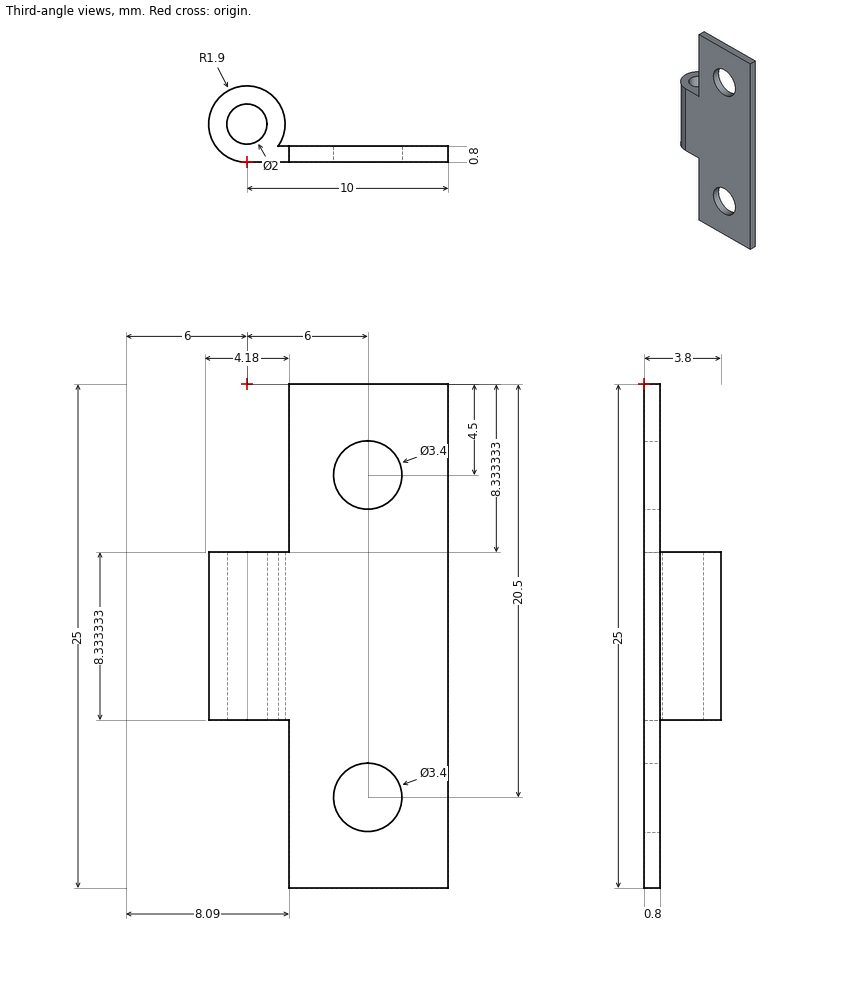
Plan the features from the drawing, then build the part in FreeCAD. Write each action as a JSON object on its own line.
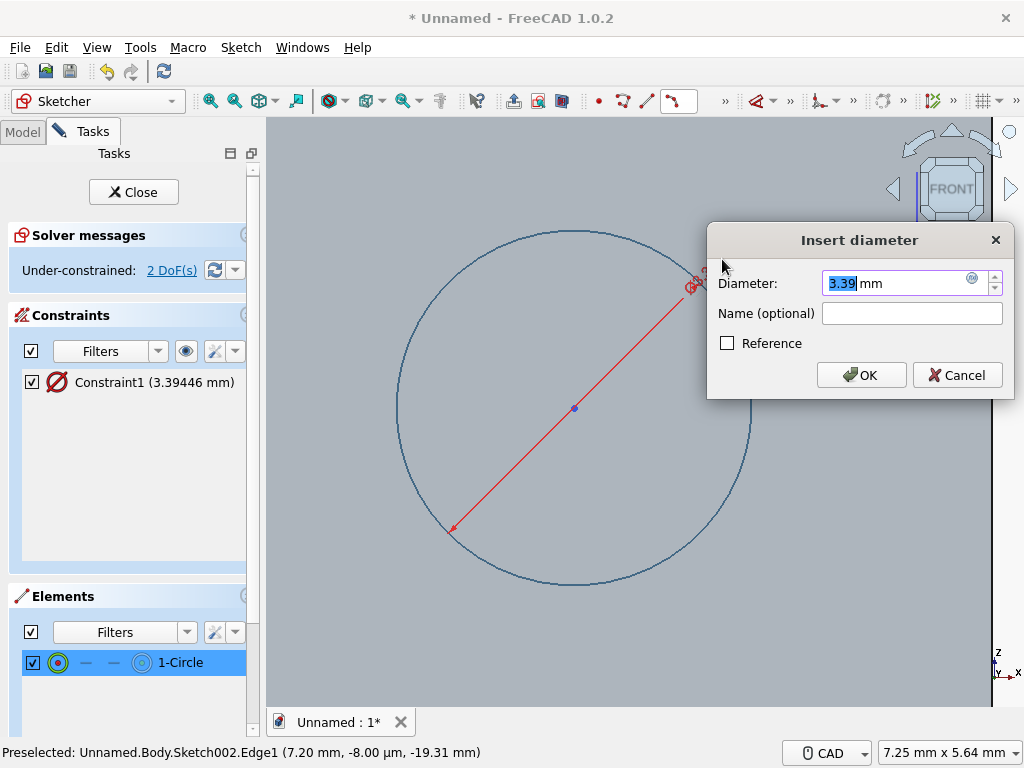
{"action": "type", "text": "3.4"}
{"action": "key", "text": "Return"}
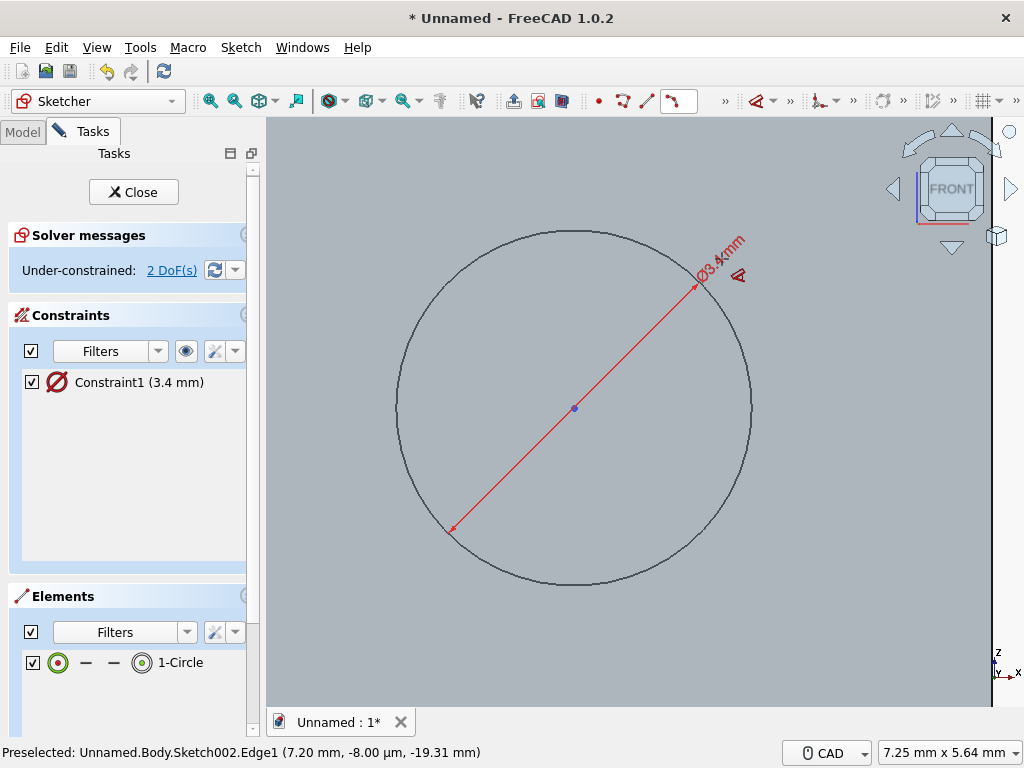
{"action": "left_click", "coordinate": [574, 408]}
{"action": "left_click", "coordinate": [434, 442]}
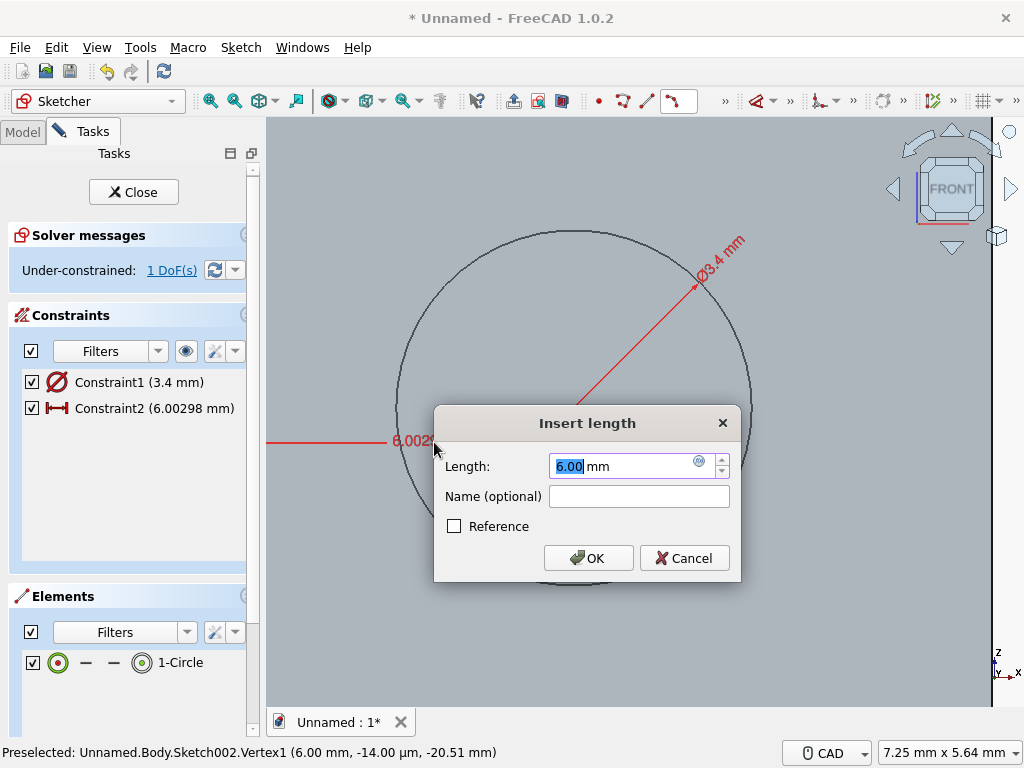
{"action": "type", "text": "6"}
{"action": "key", "text": "Return"}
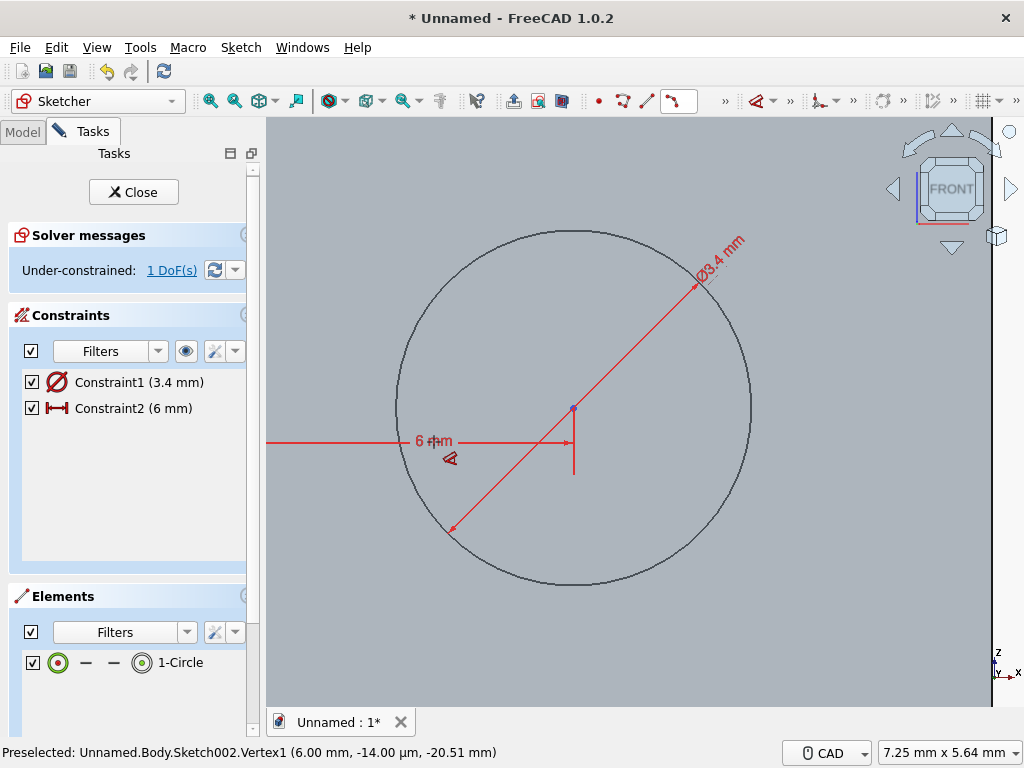
{"action": "left_click", "coordinate": [574, 408]}
{"action": "left_click", "coordinate": [608, 277]}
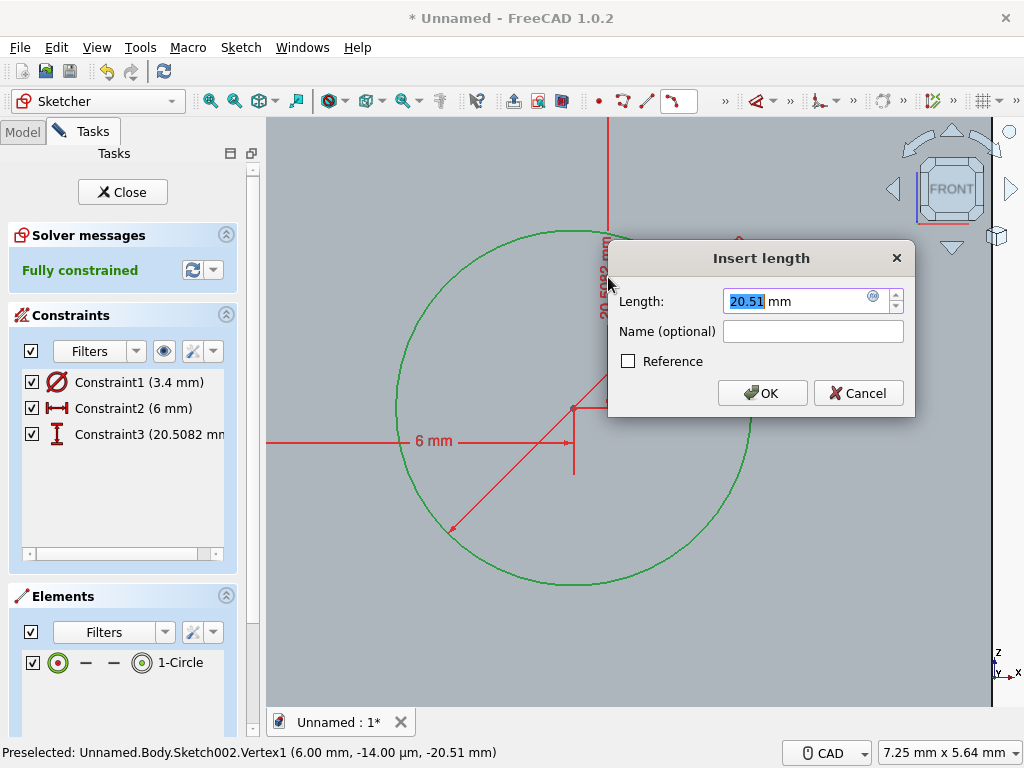
{"action": "type", "text": "20.5"}
{"action": "key", "text": "Return"}
{"action": "key", "text": "Escape"}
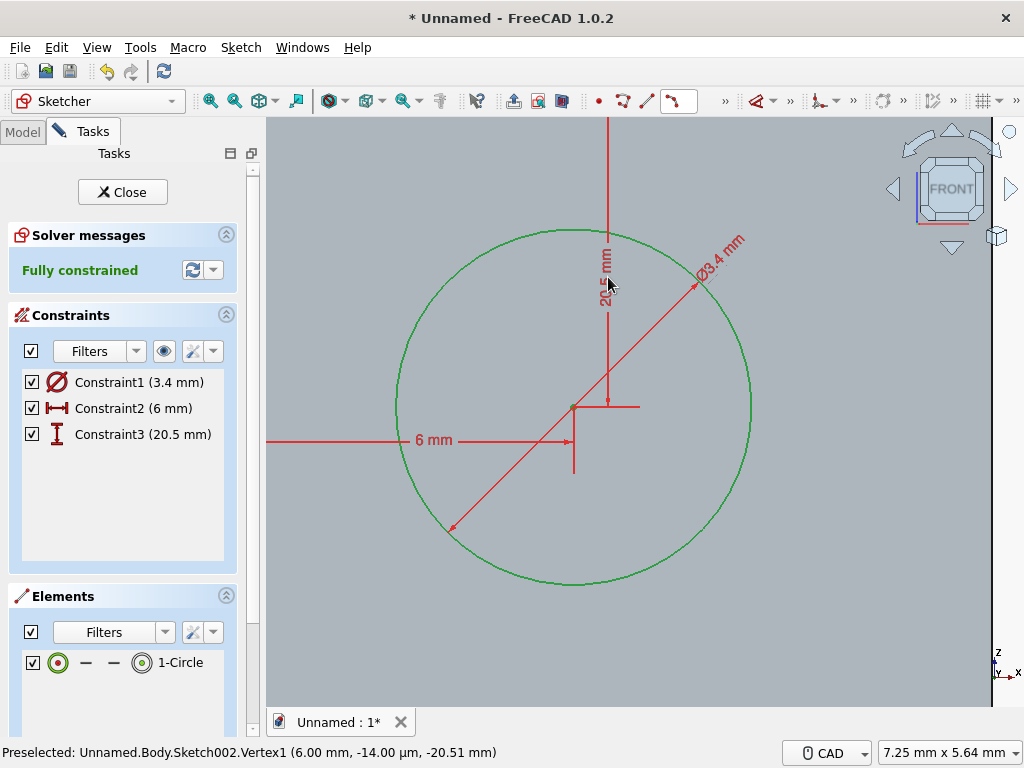
{"action": "left_click", "coordinate": [123, 192]}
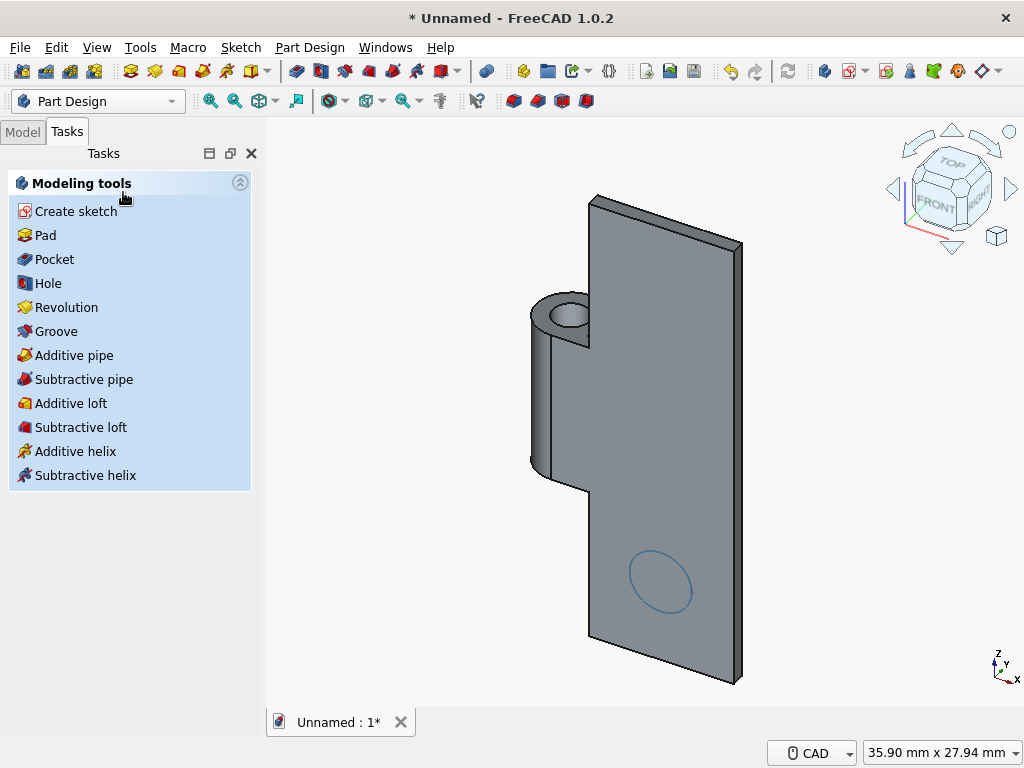
{"action": "left_click", "coordinate": [298, 72]}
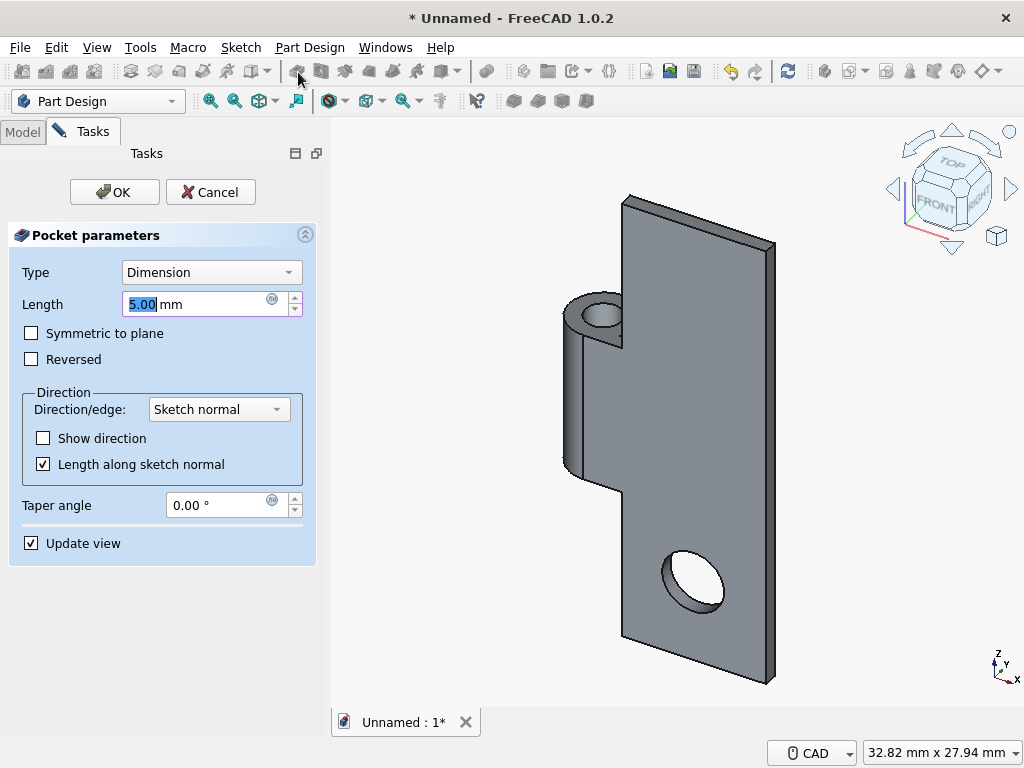
{"action": "type", "text": "0.8"}
{"action": "key", "text": "Tab"}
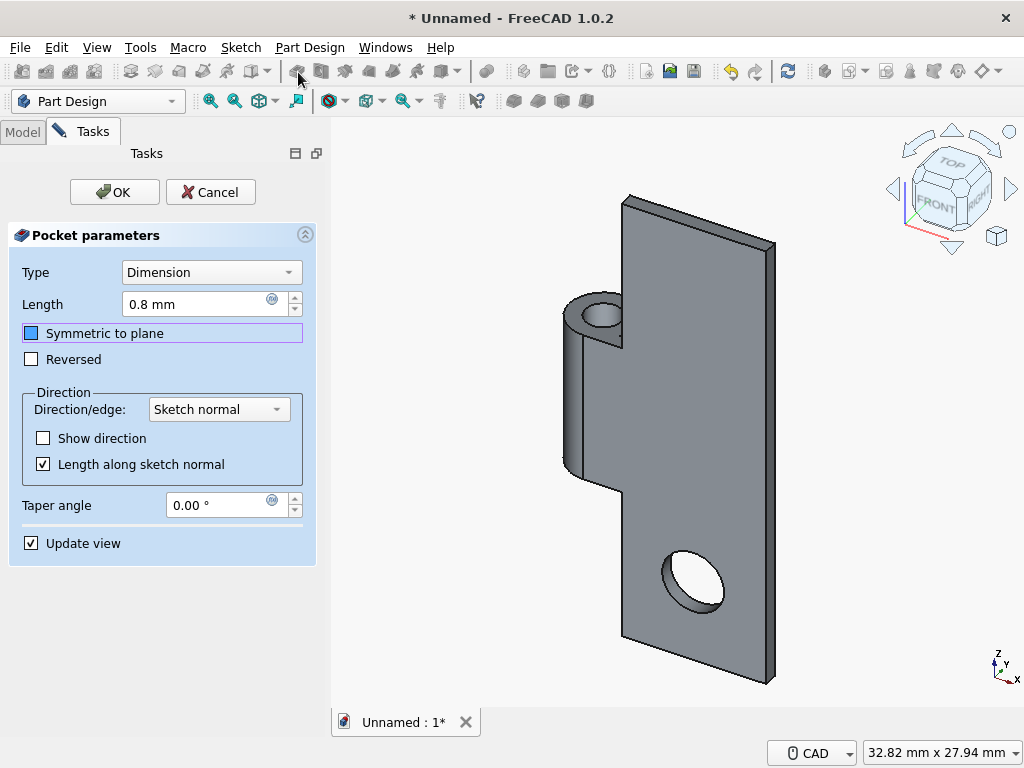
{"action": "left_click", "coordinate": [115, 192]}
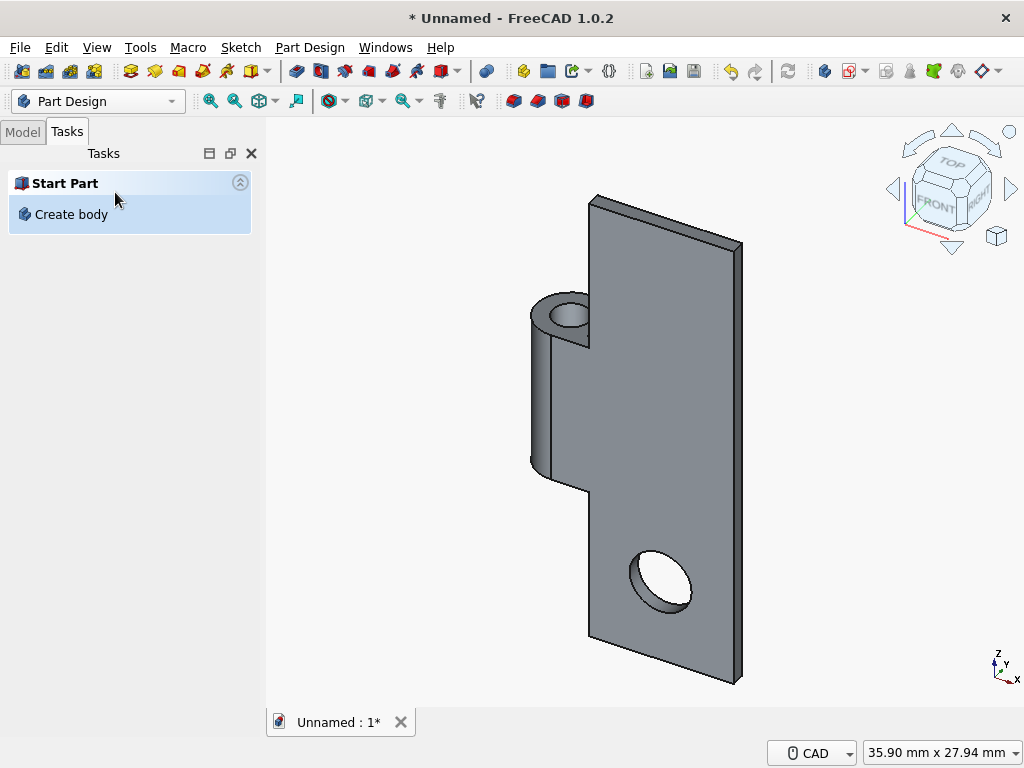
{"action": "left_click", "coordinate": [850, 72]}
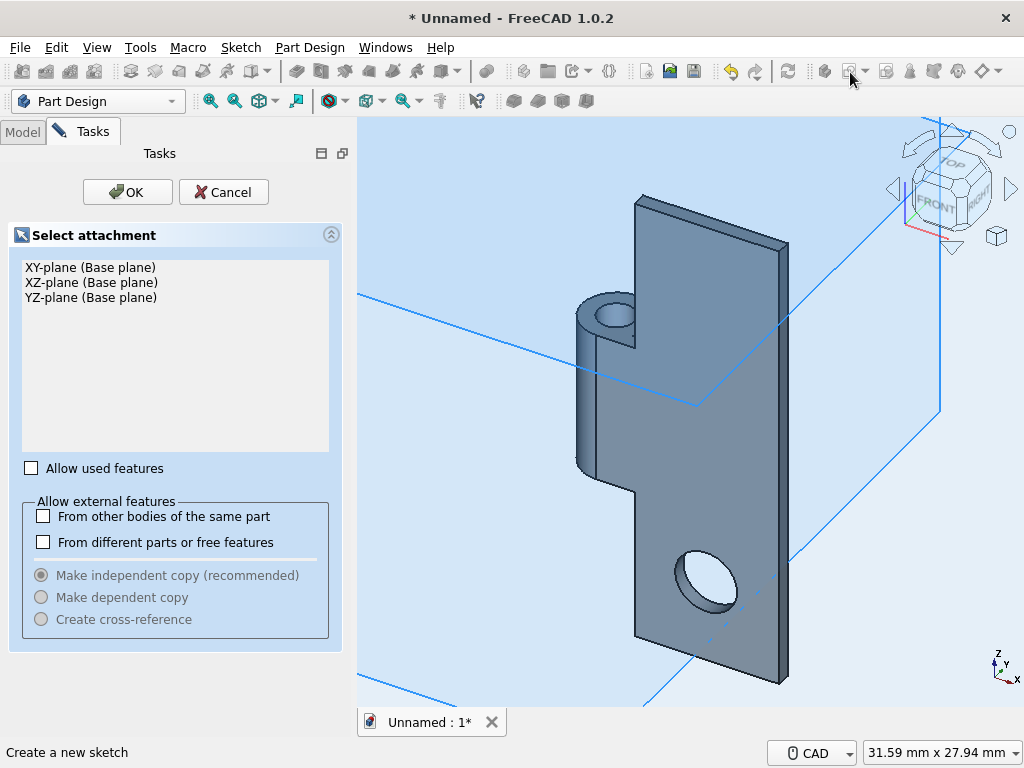
{"action": "left_click", "coordinate": [82, 282]}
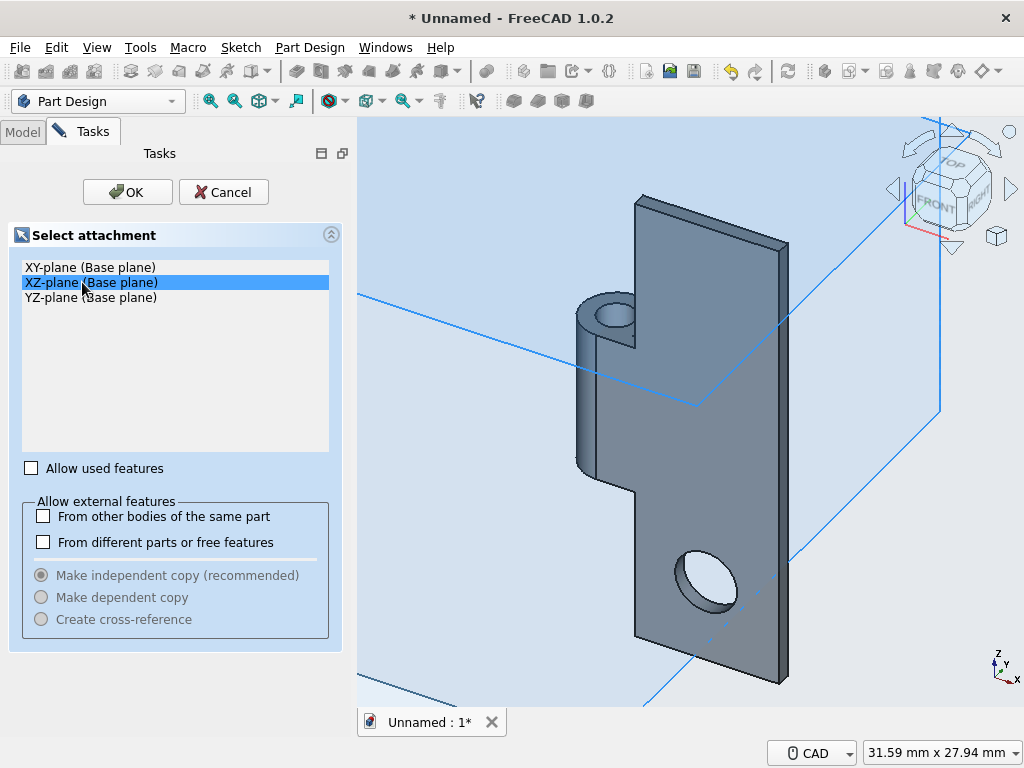
{"action": "left_click", "coordinate": [128, 192]}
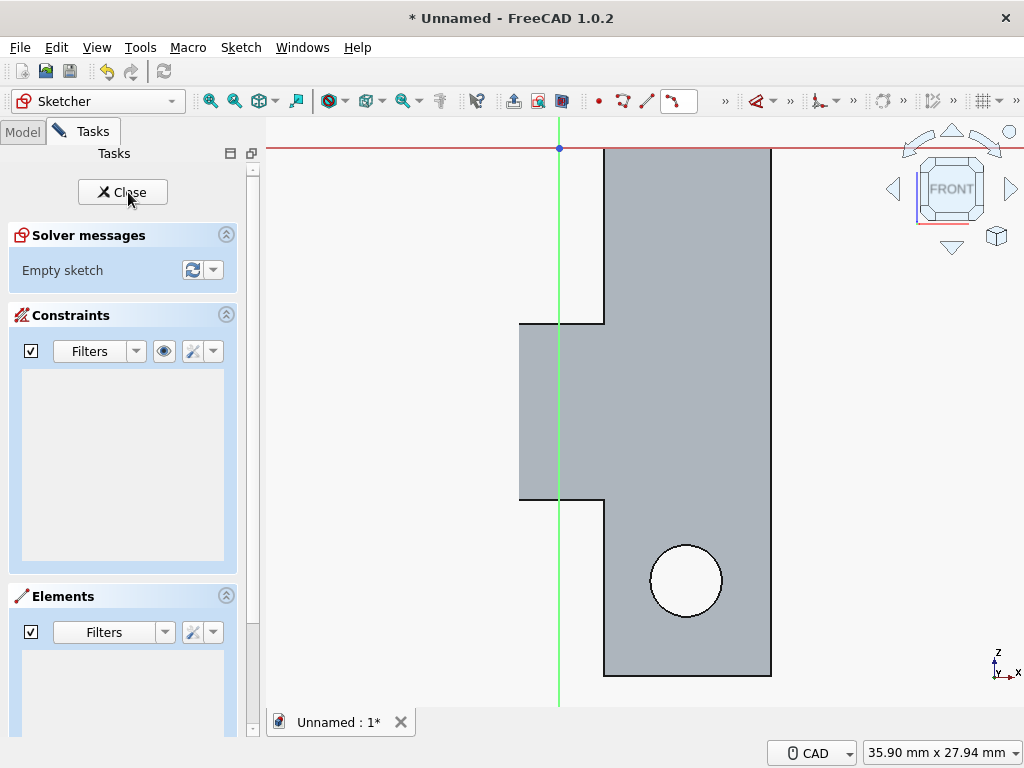
{"action": "scroll", "coordinate": [576, 412], "scroll_direction": "down", "scroll_amount": 5}